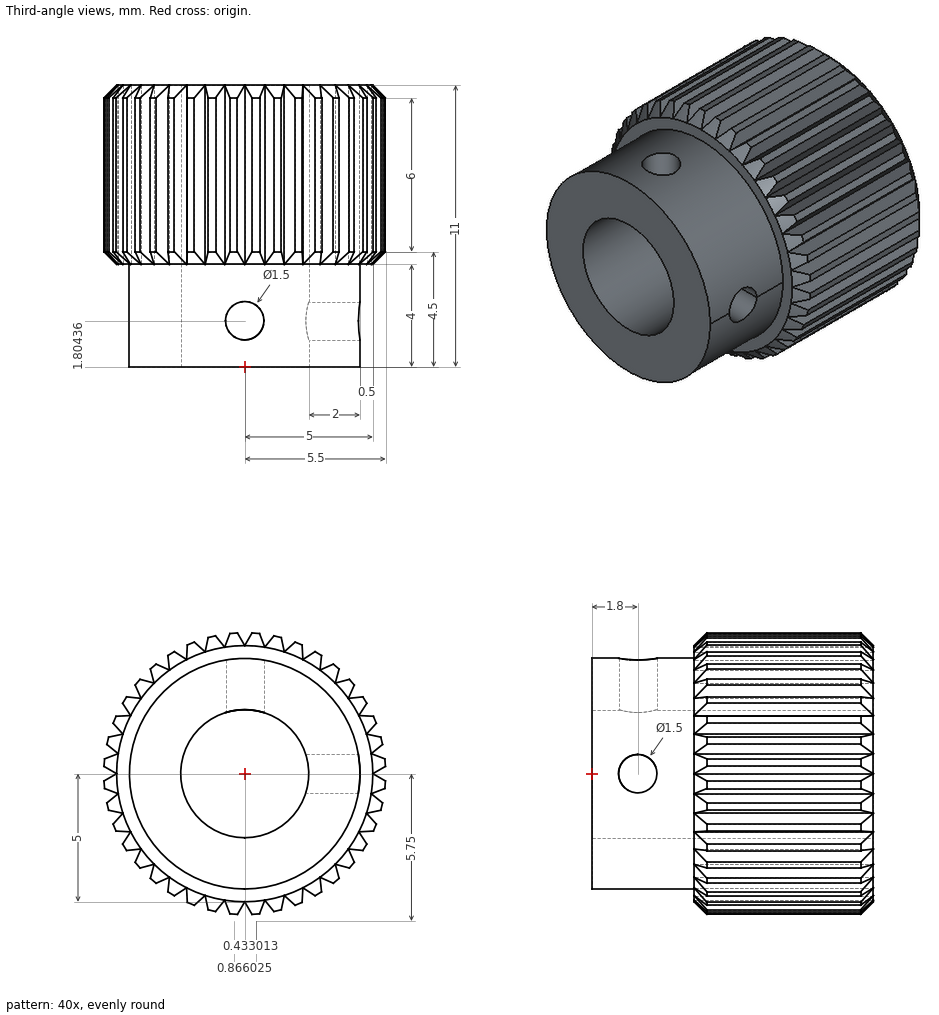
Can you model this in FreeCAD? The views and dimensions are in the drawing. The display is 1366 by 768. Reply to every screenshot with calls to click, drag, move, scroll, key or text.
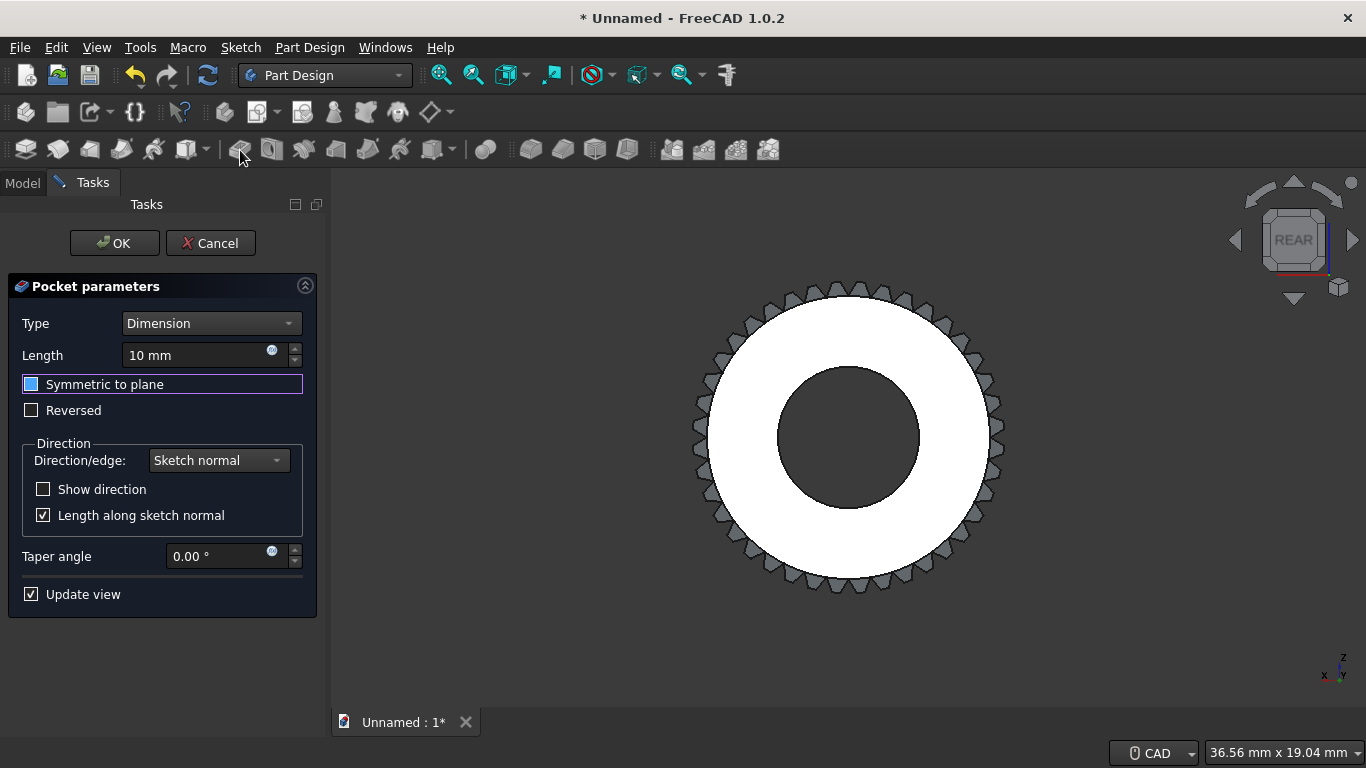
click(30, 410)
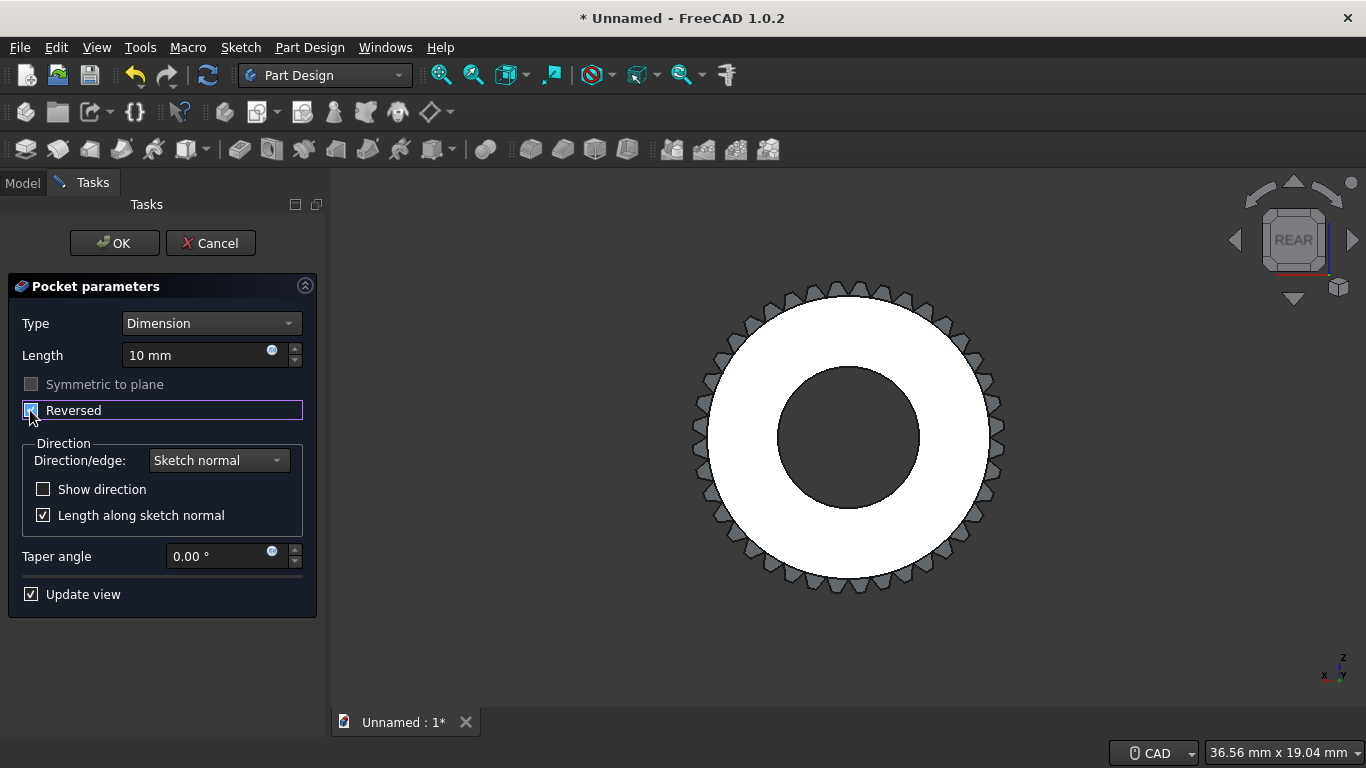
click(115, 243)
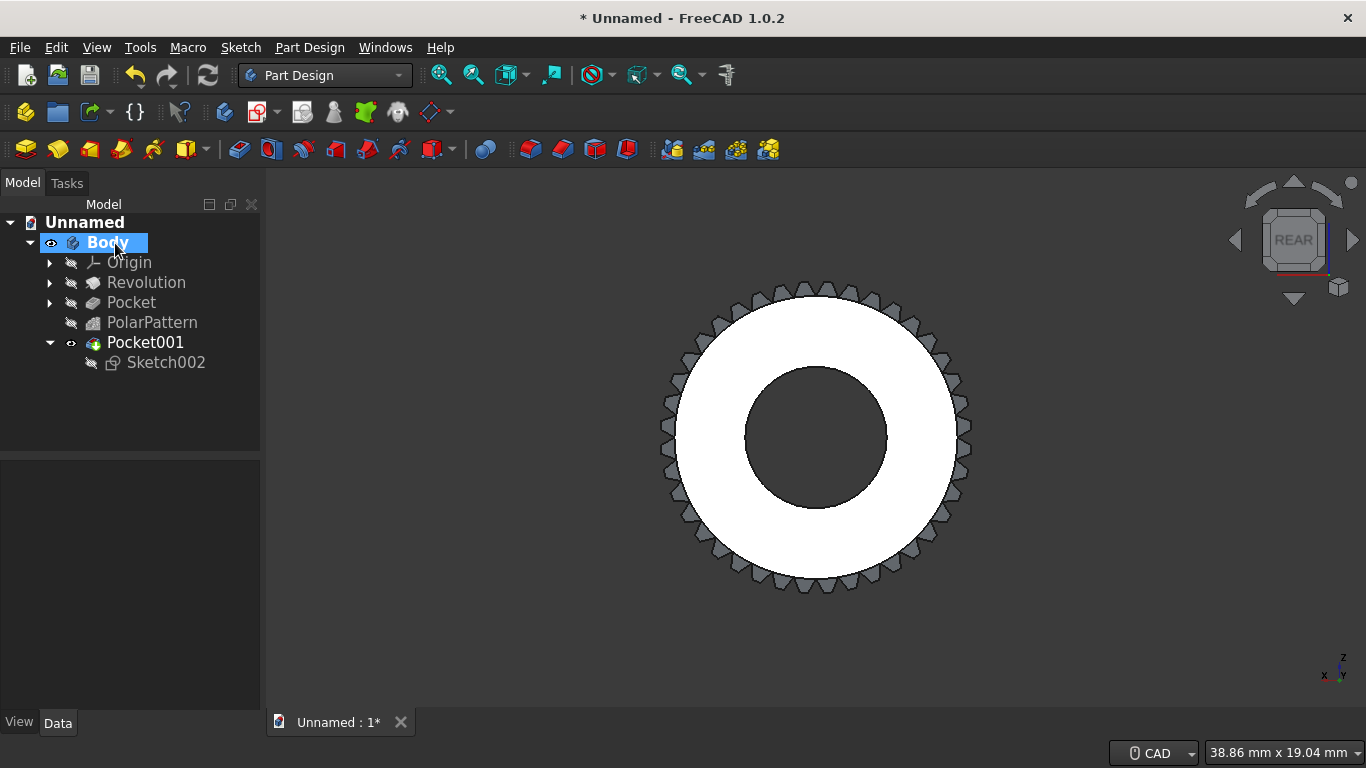
click(258, 112)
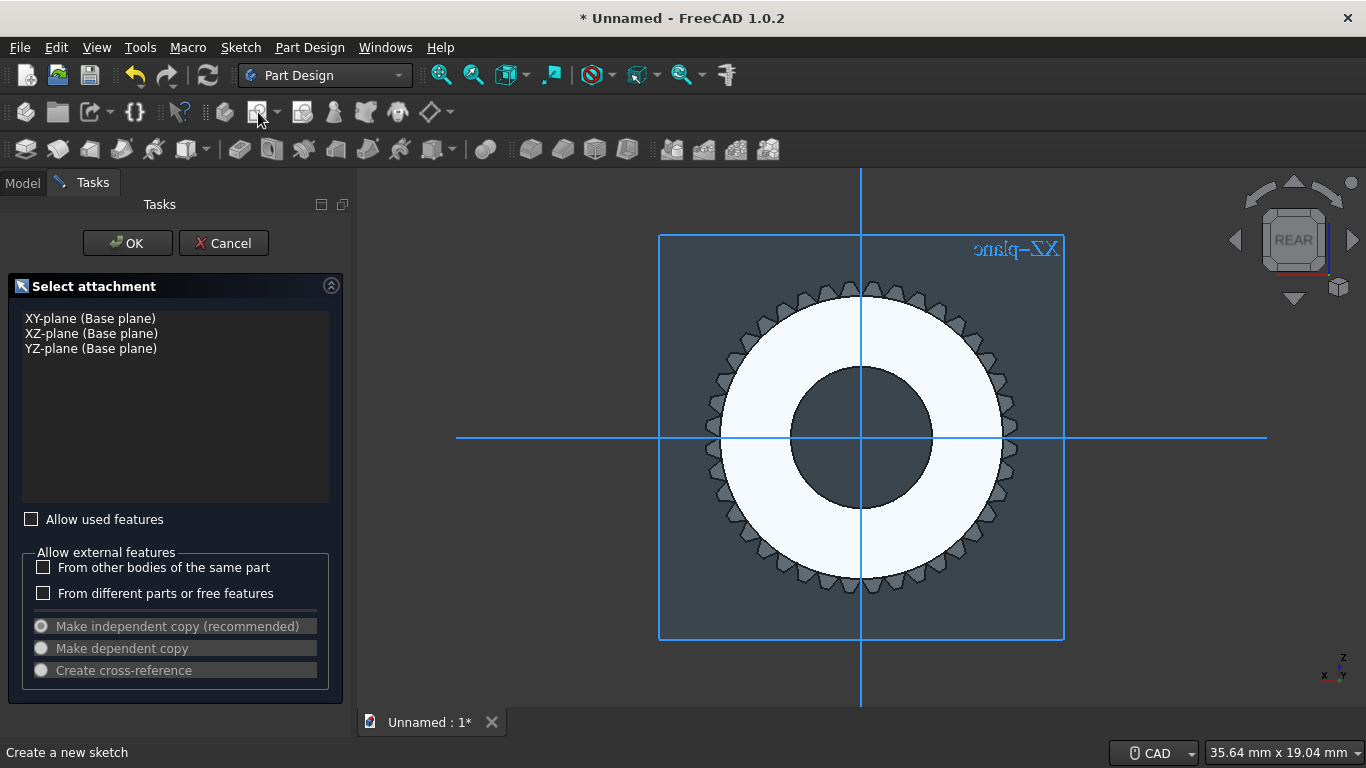
click(82, 348)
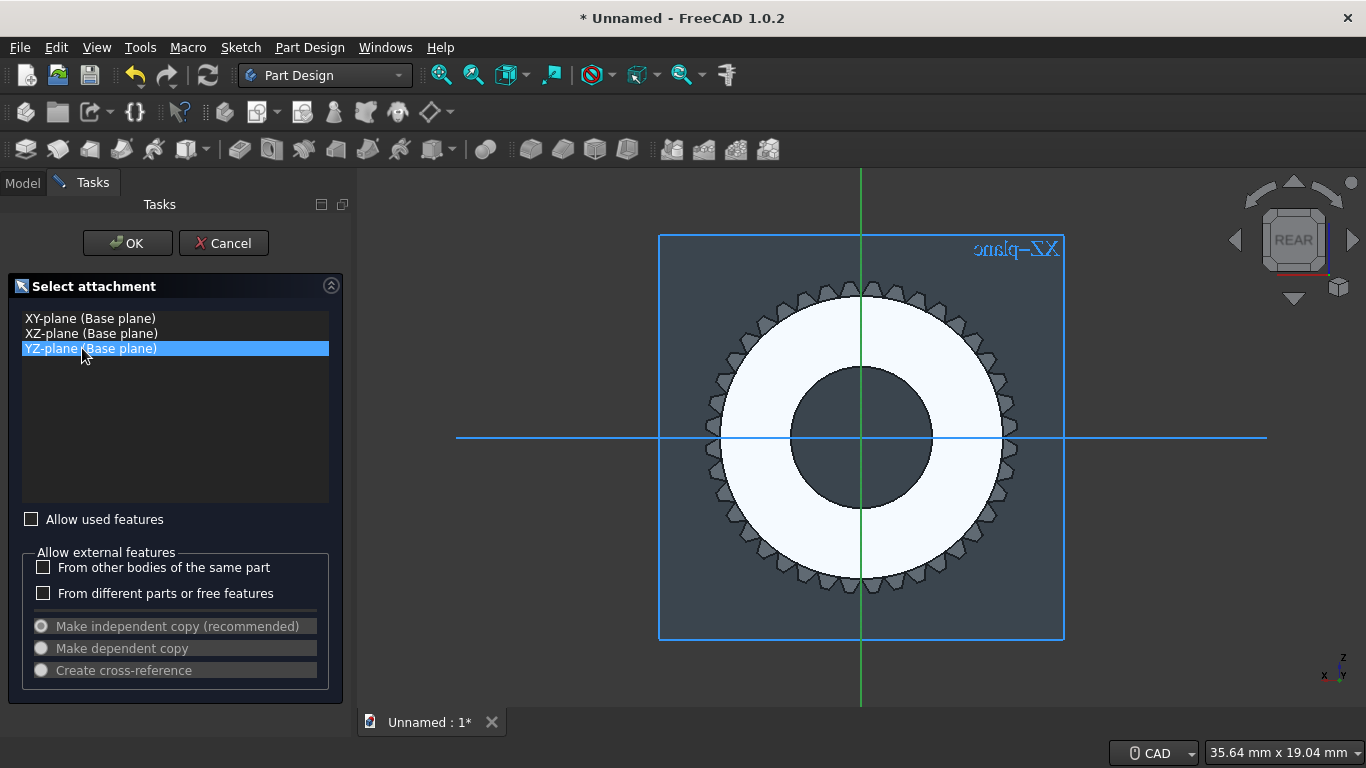
click(128, 243)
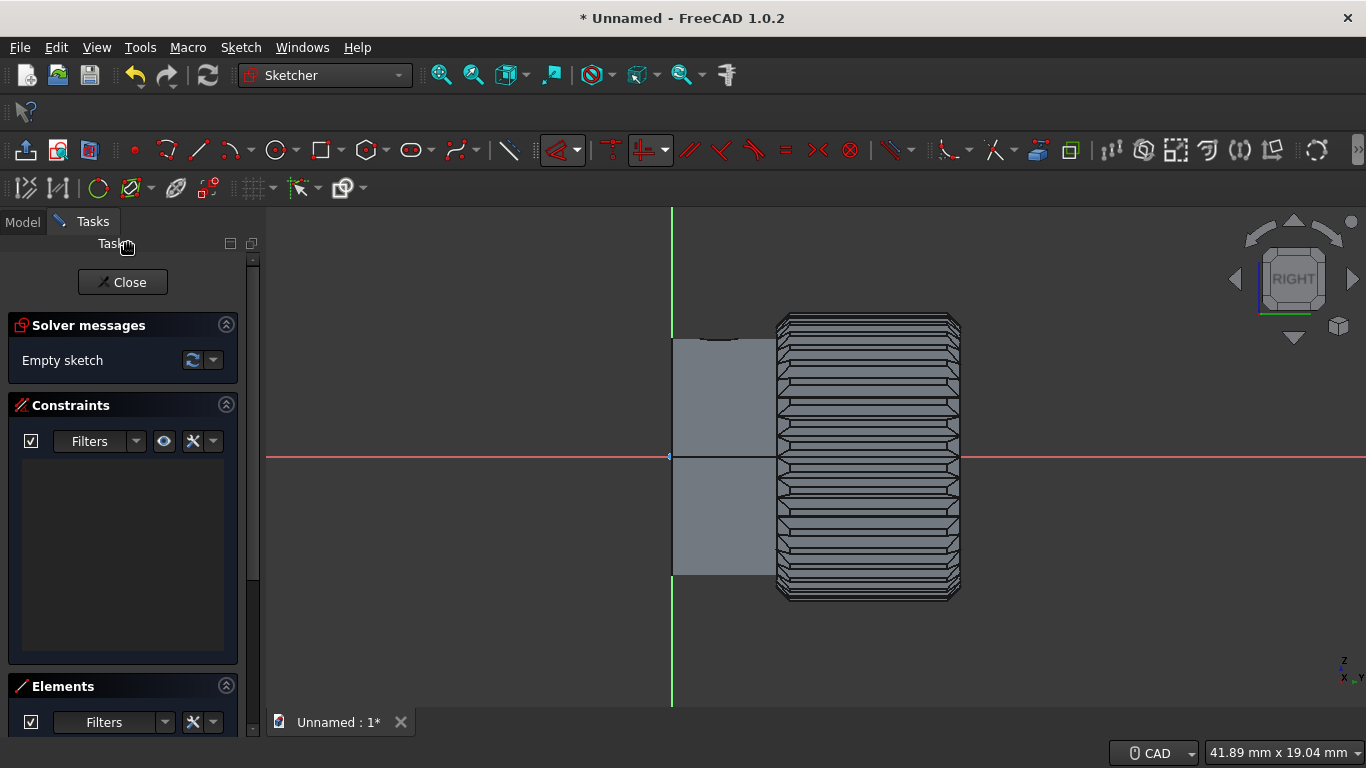
key(q)
key(s)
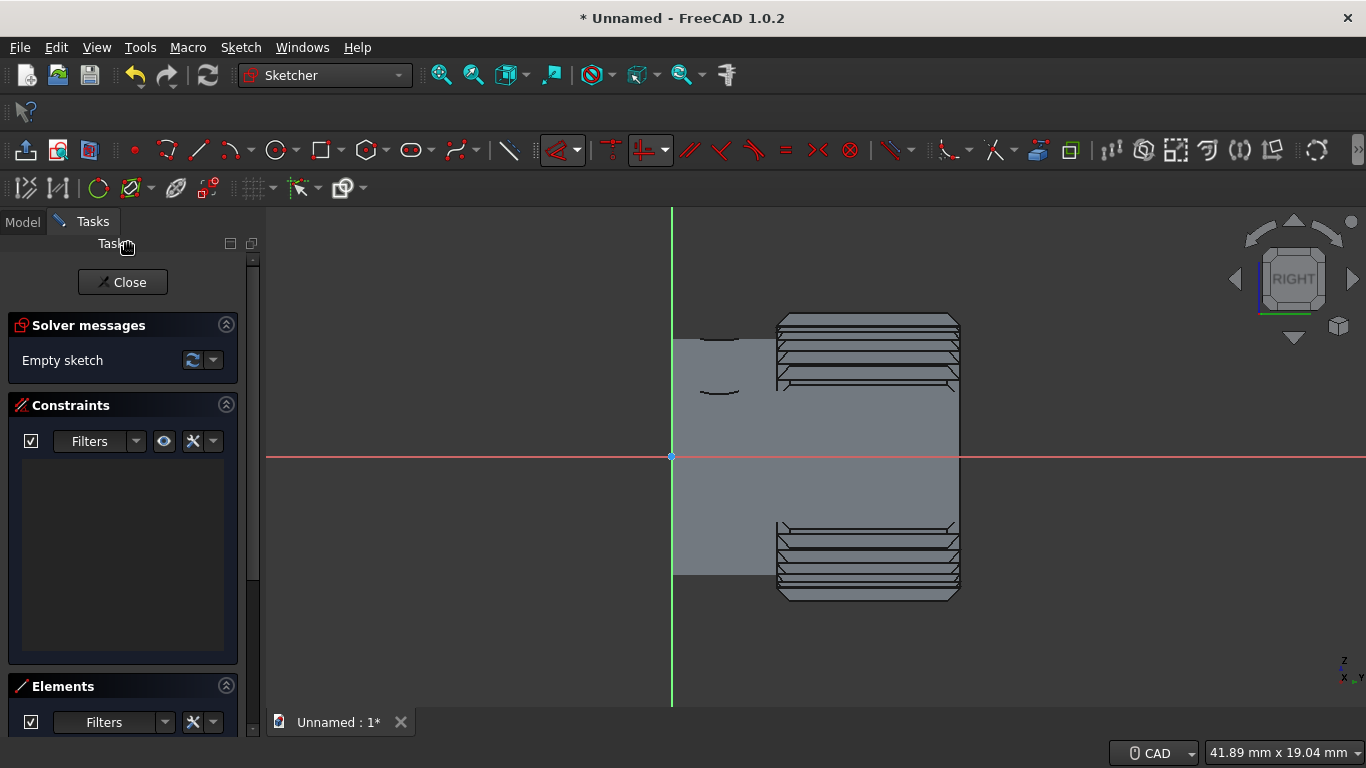
scroll(698, 457, up, 10)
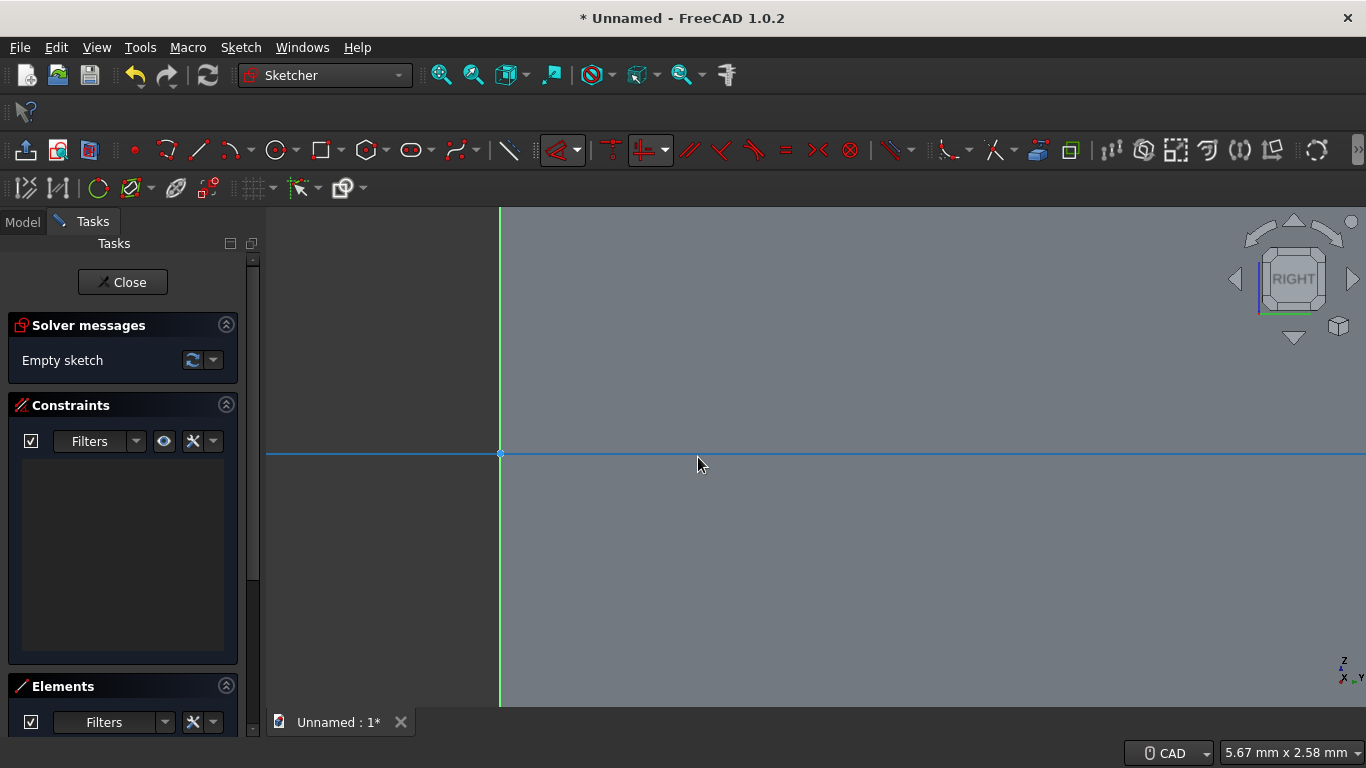
key(g)
key(c)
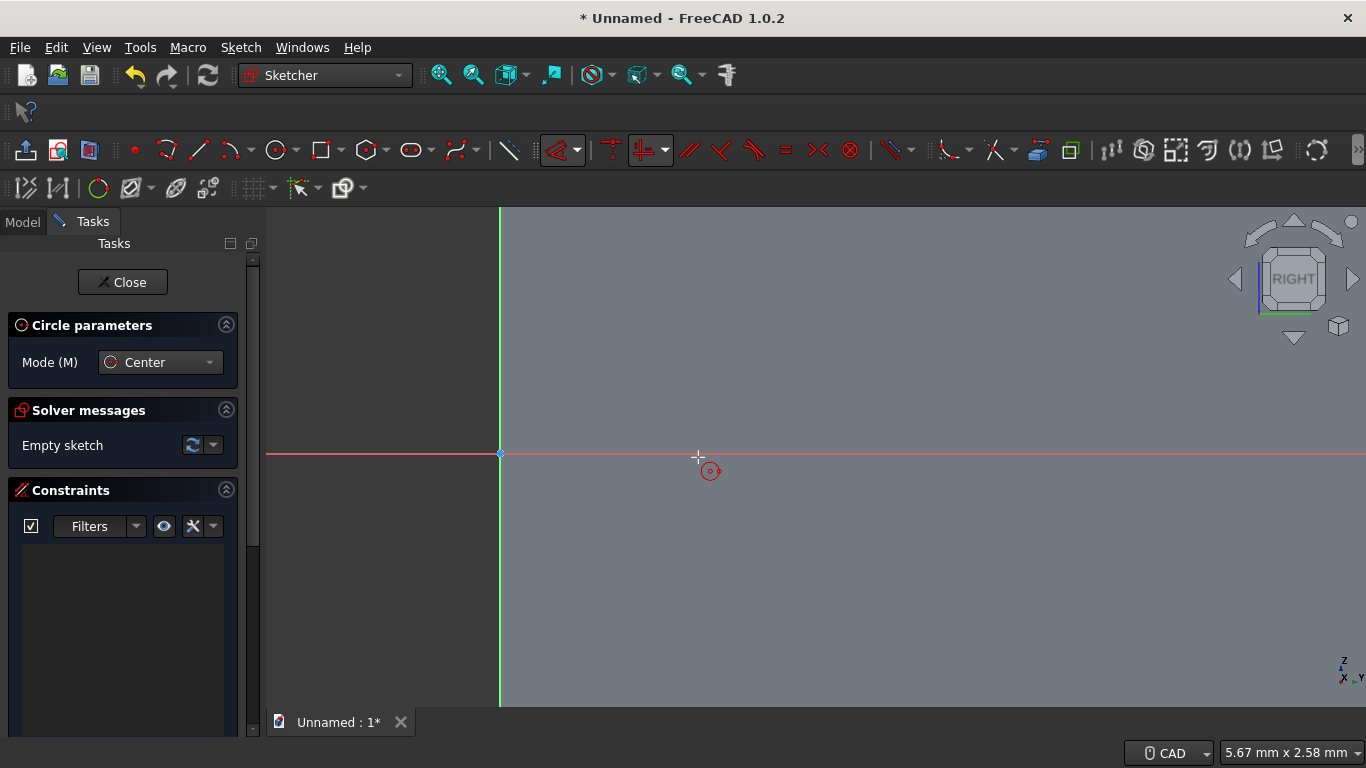
click(849, 454)
move(952, 351)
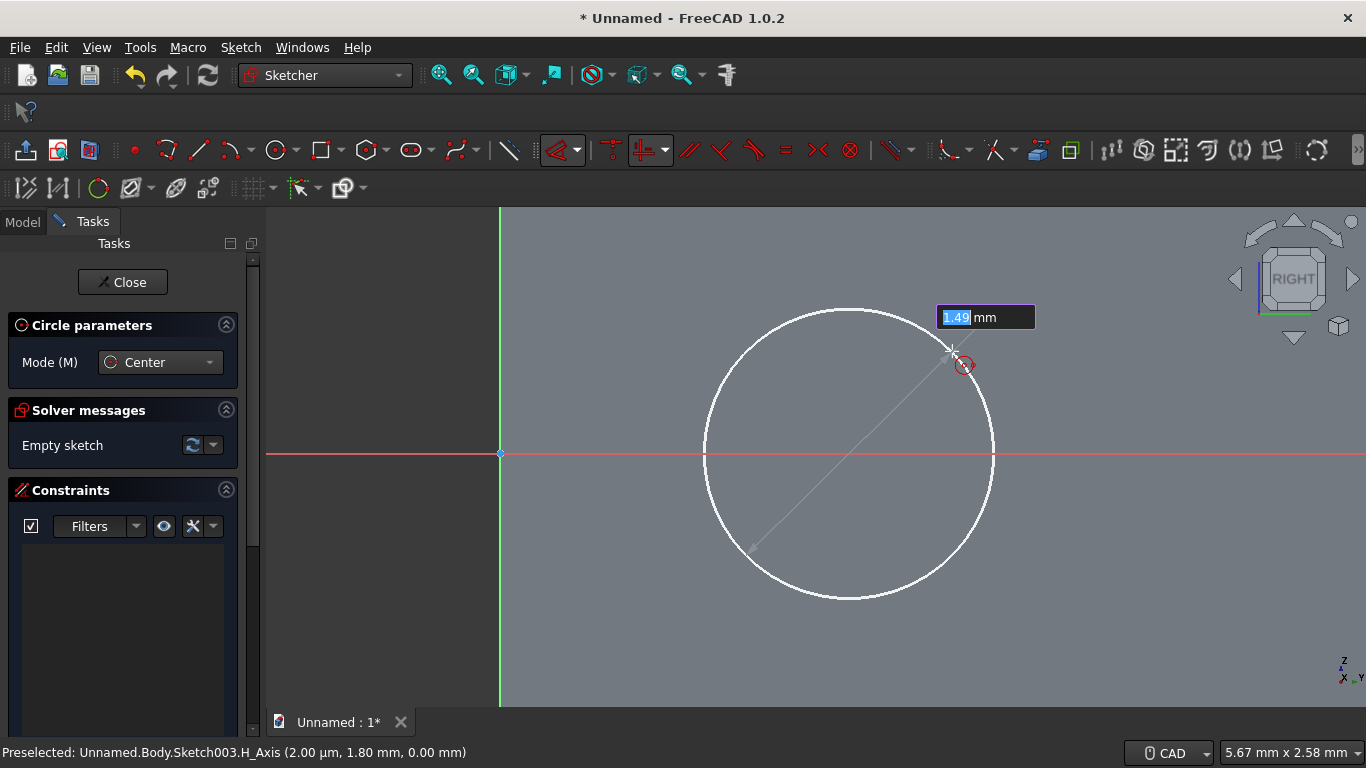
text(1.5)
key(Return)
key(Escape)